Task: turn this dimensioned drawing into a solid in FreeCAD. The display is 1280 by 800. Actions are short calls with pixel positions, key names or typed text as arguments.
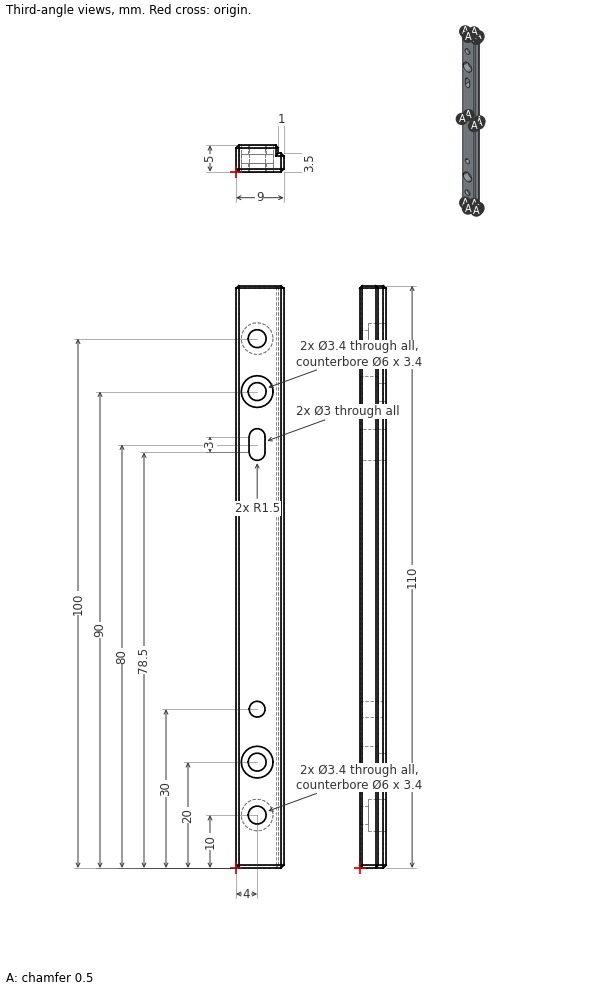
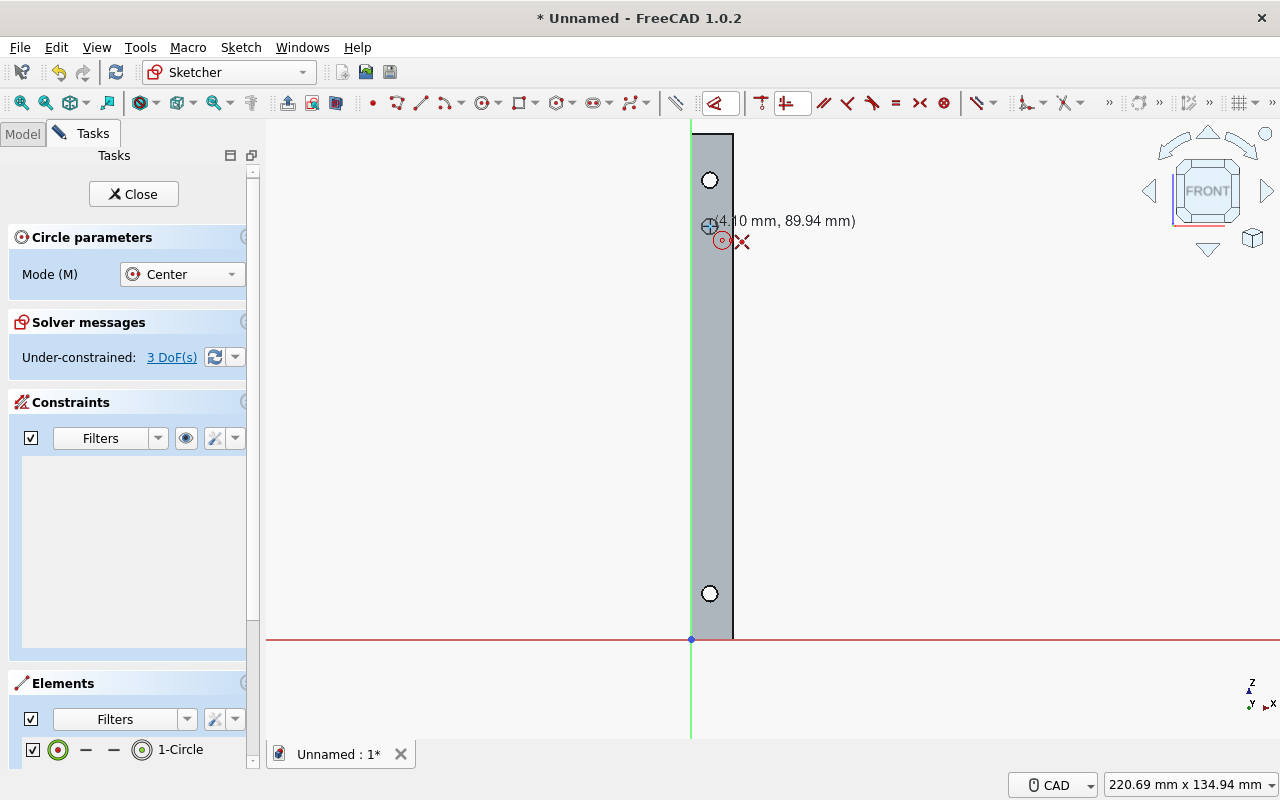
scroll(710, 548, up, 6)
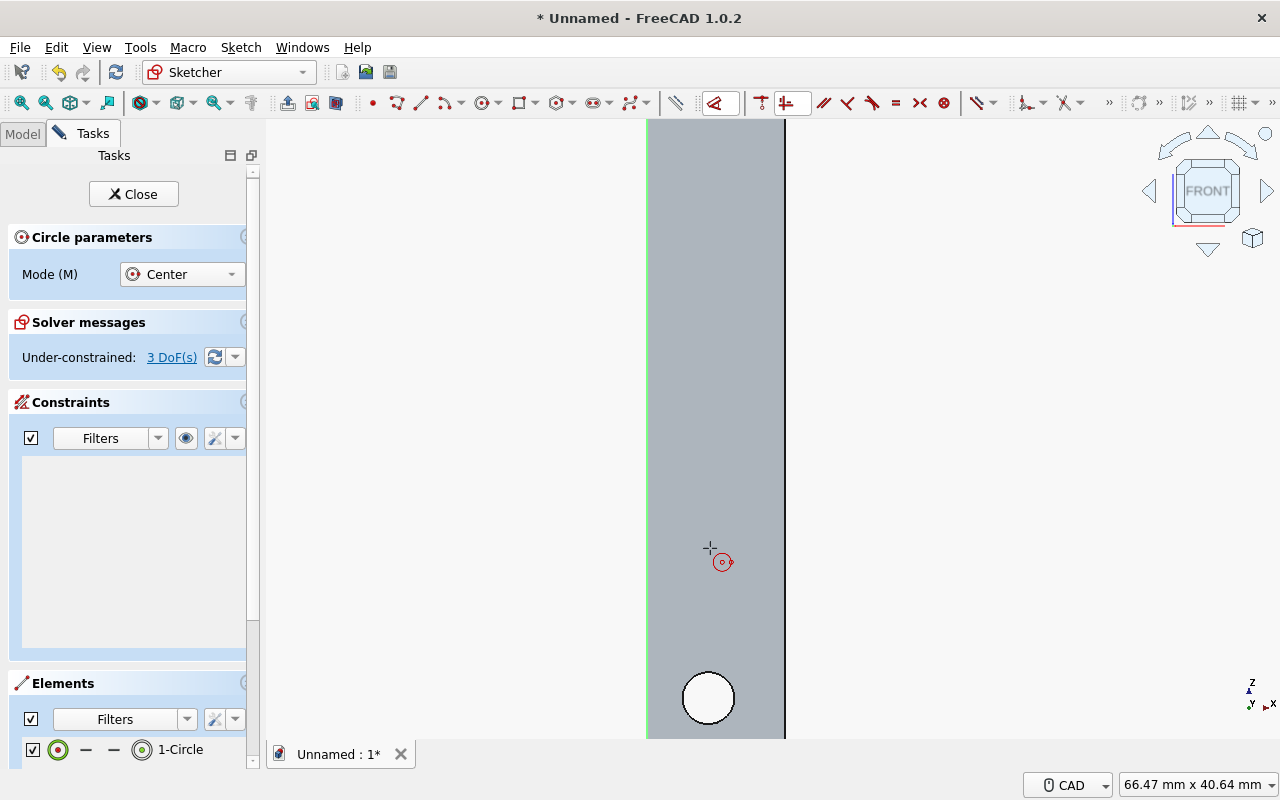
click(708, 546)
click(727, 527)
key(Escape)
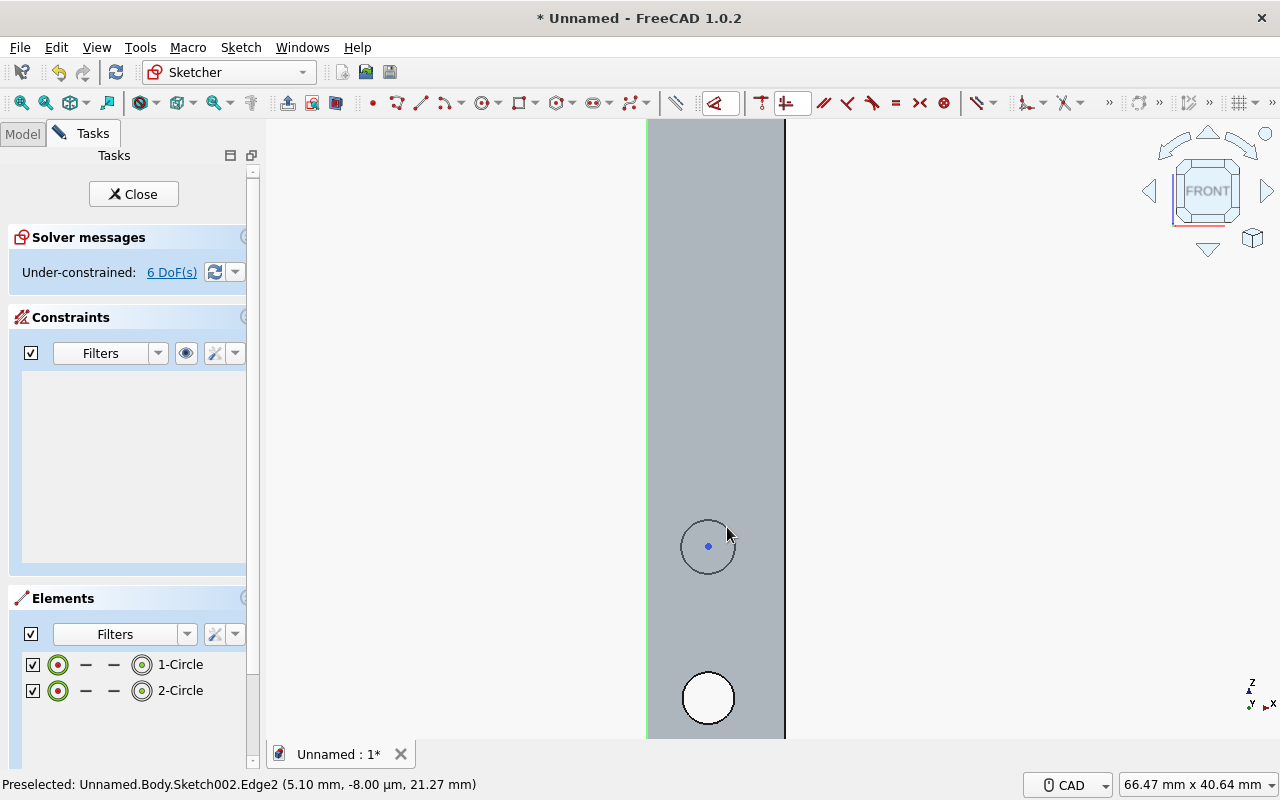
scroll(710, 549, down, 6)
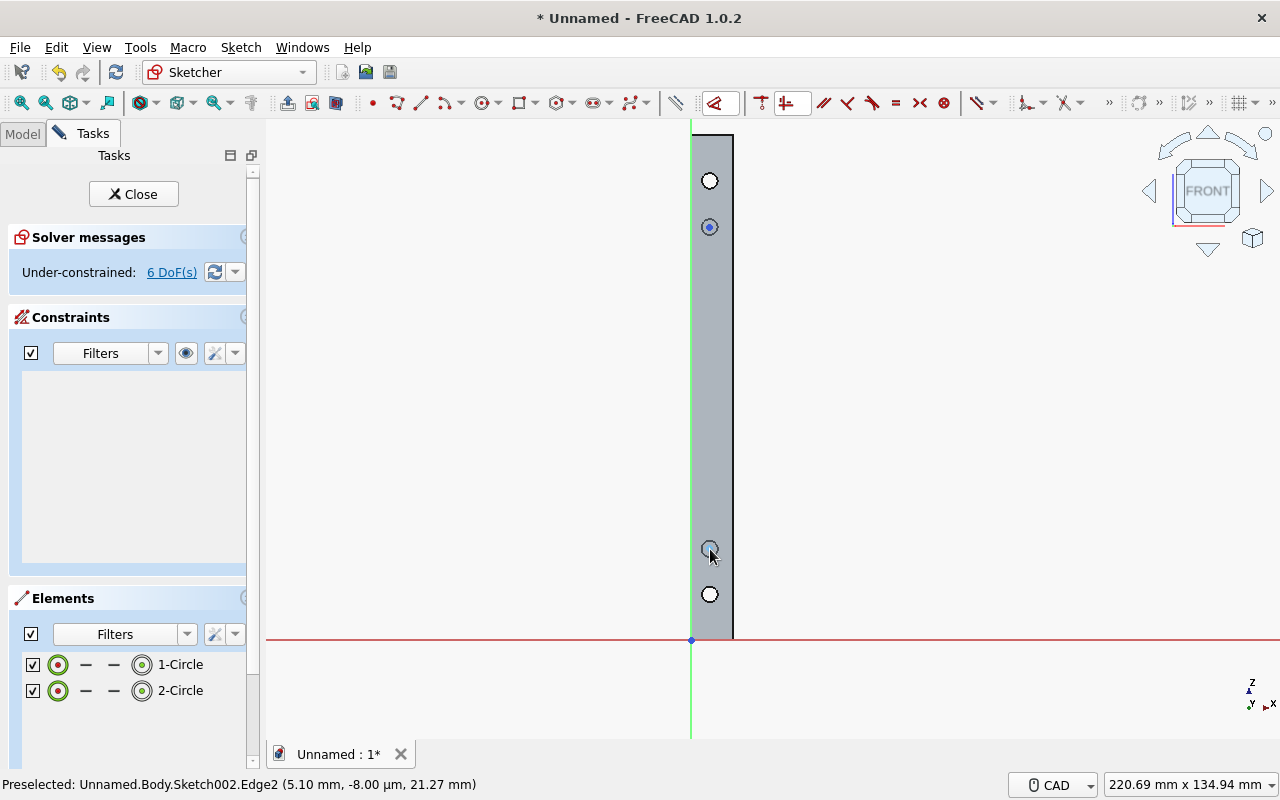
scroll(715, 222, up, 3)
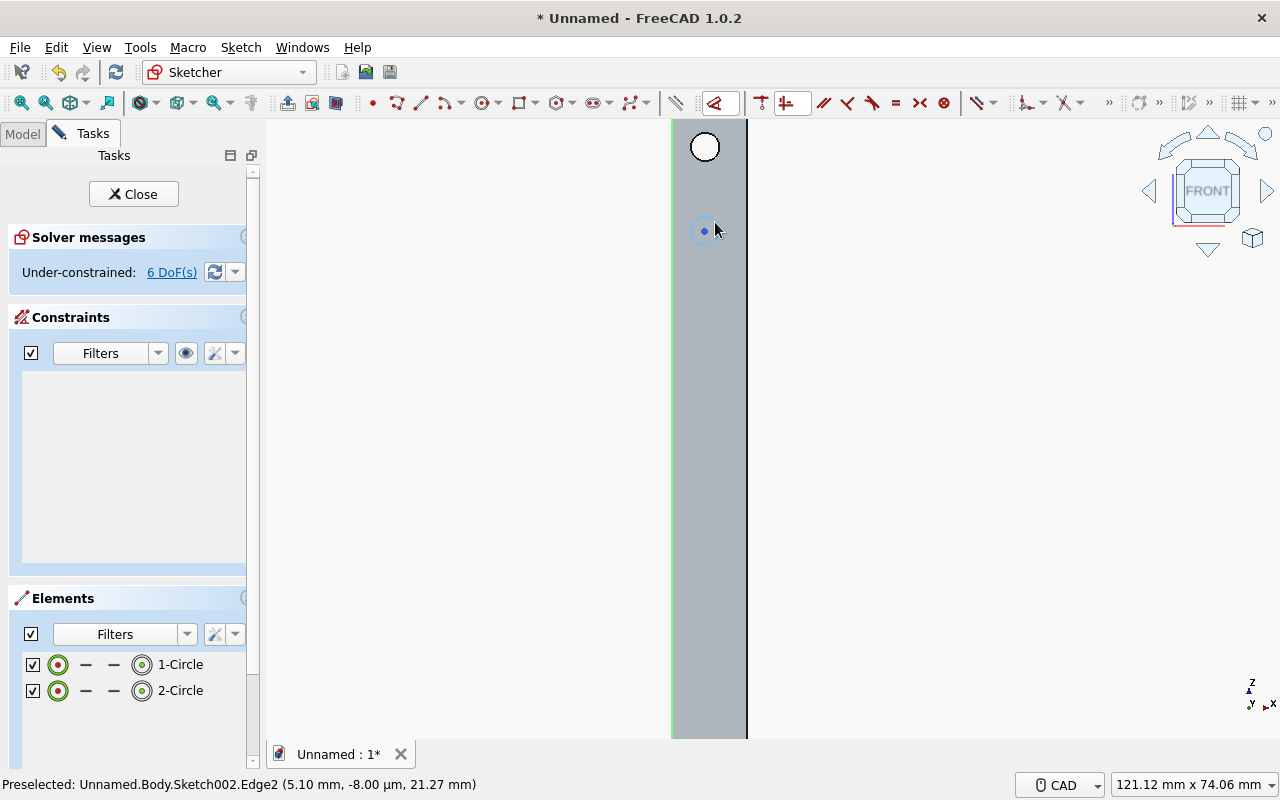
click(715, 221)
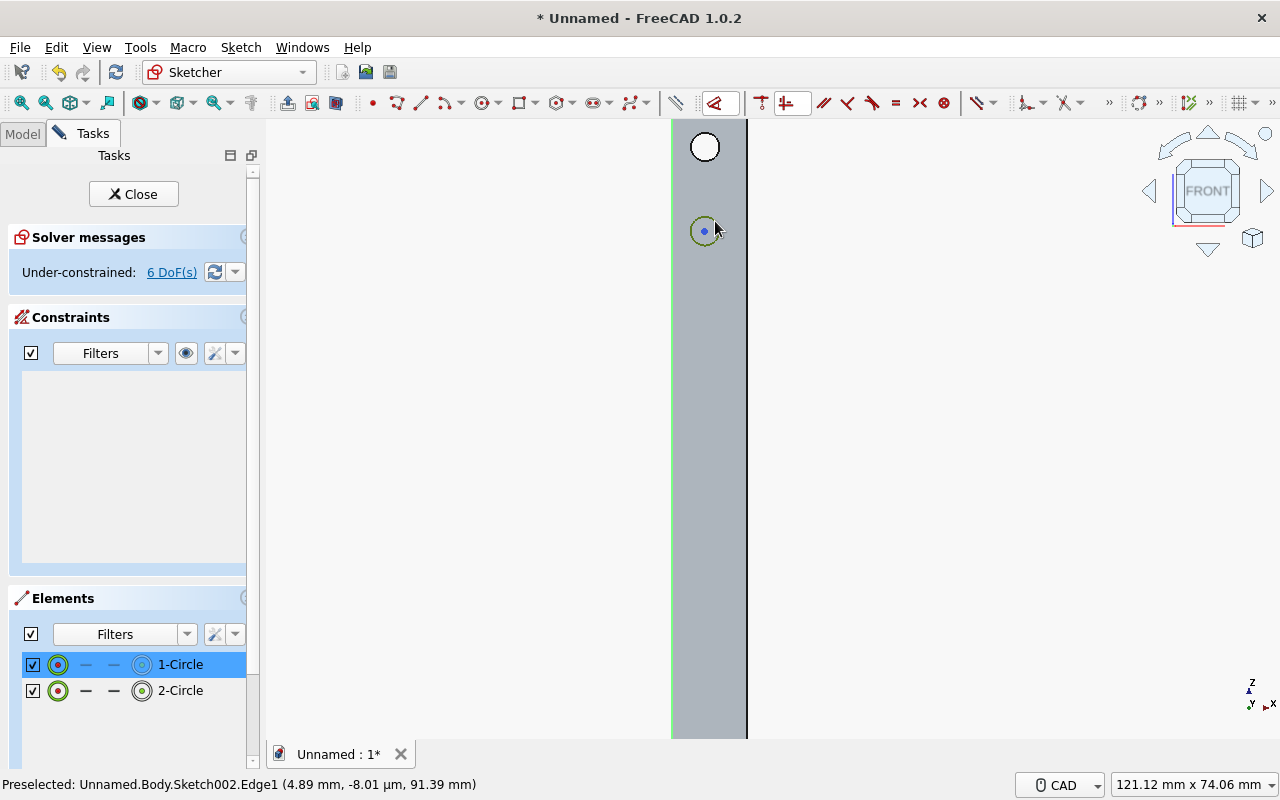
scroll(715, 221, down, 3)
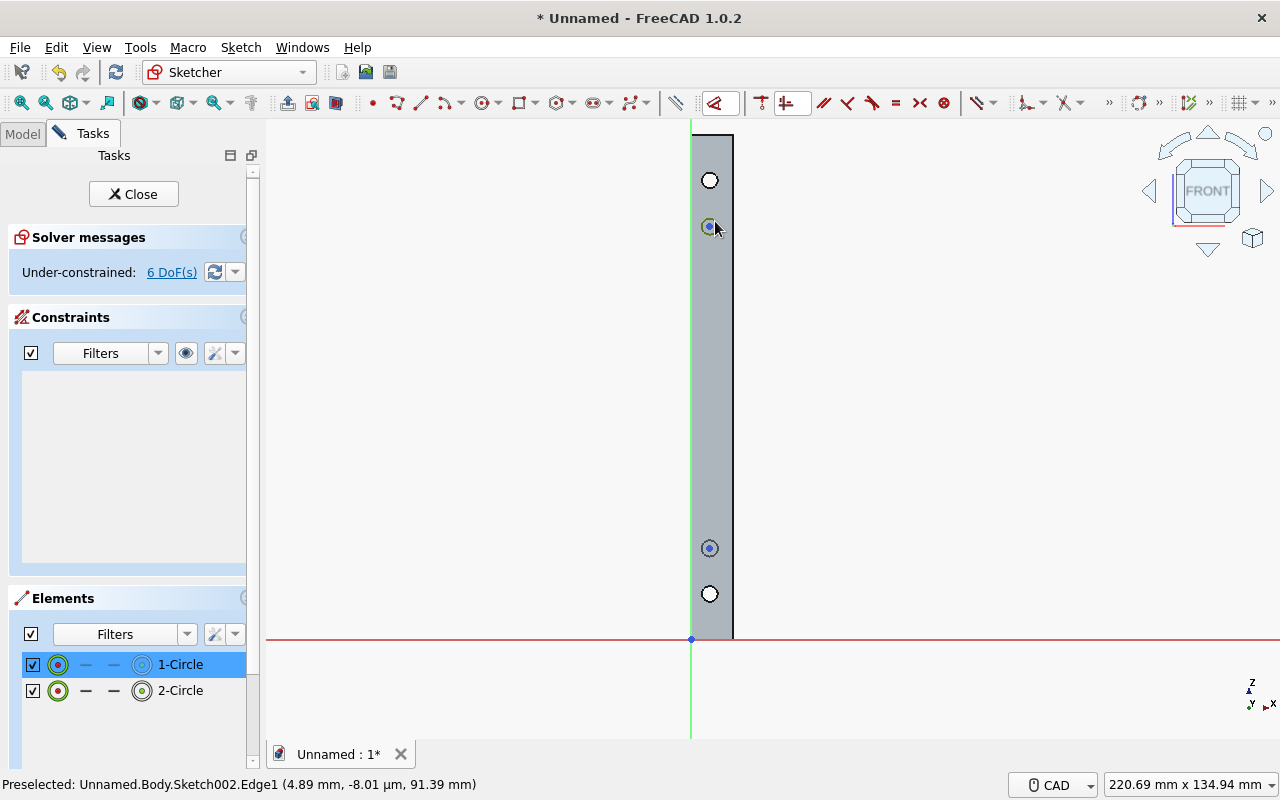
scroll(715, 543, up, 3)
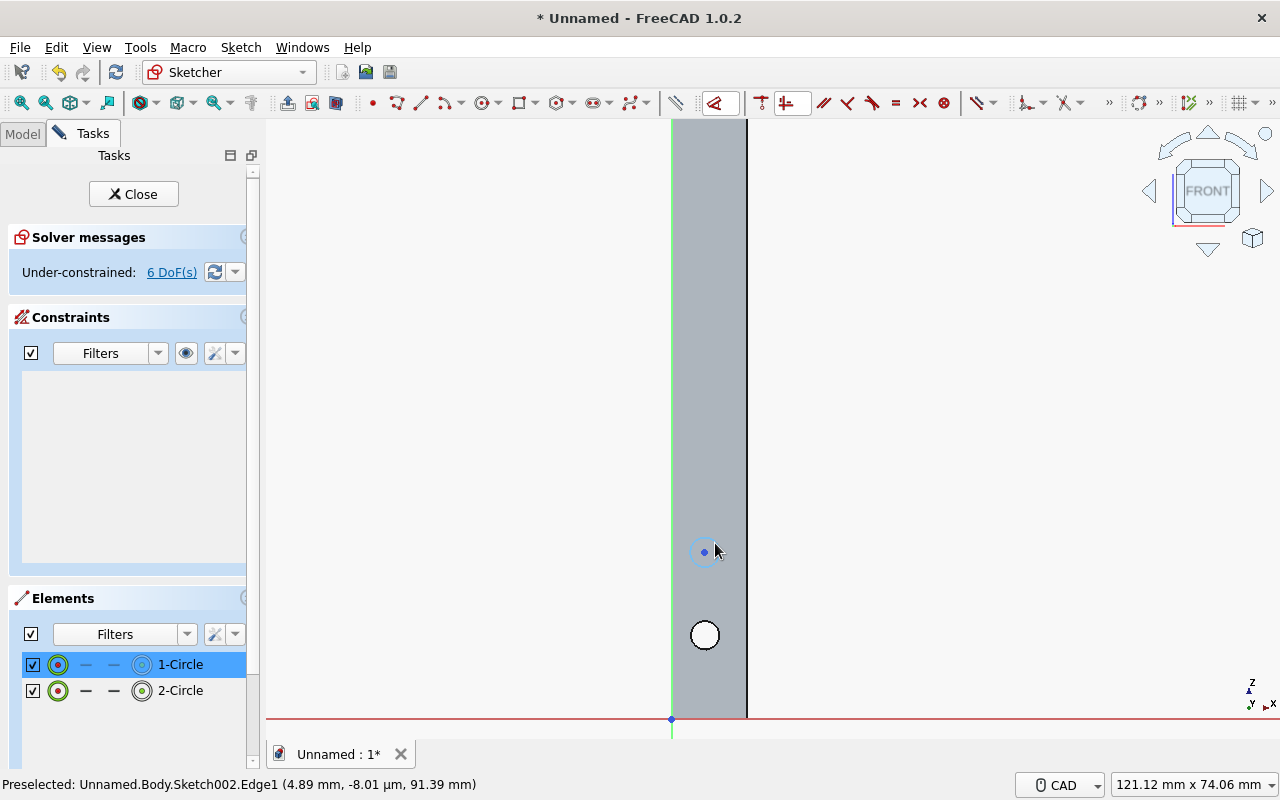
click(715, 542)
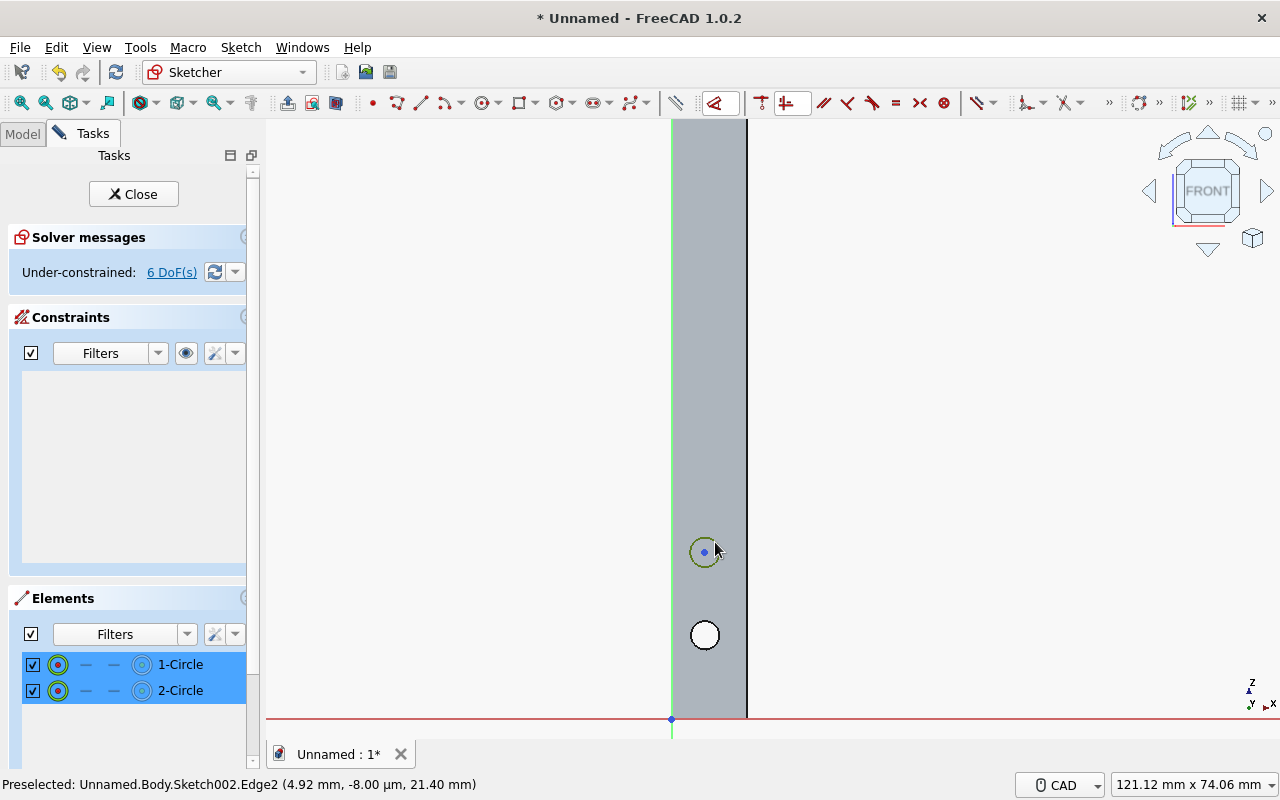
click(896, 104)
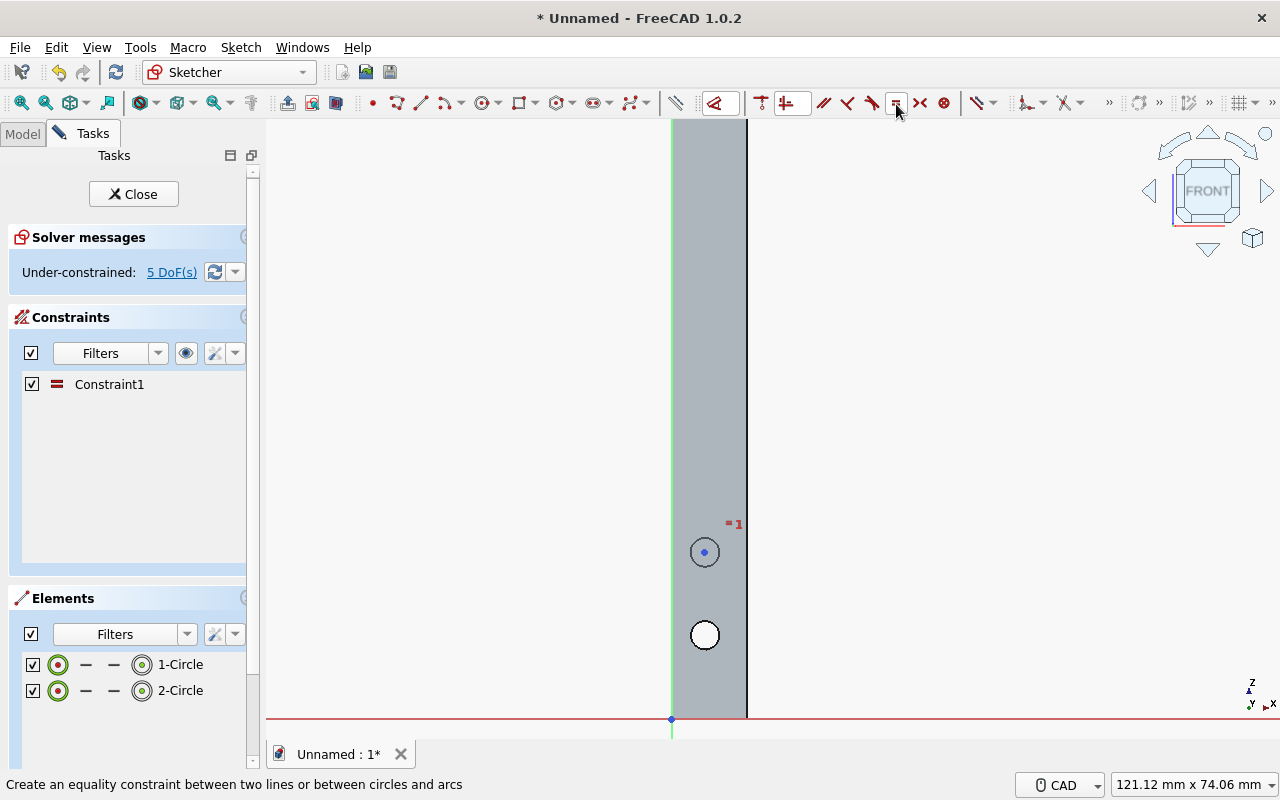
key(d)